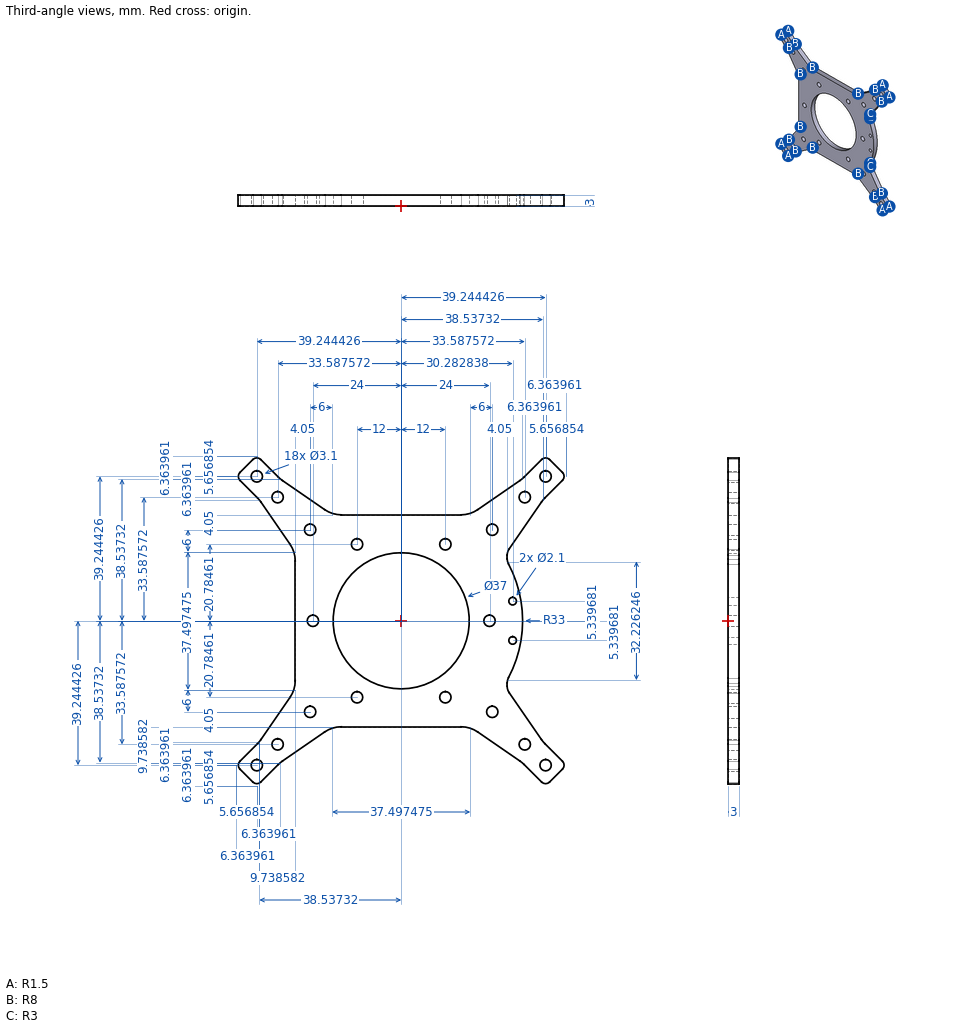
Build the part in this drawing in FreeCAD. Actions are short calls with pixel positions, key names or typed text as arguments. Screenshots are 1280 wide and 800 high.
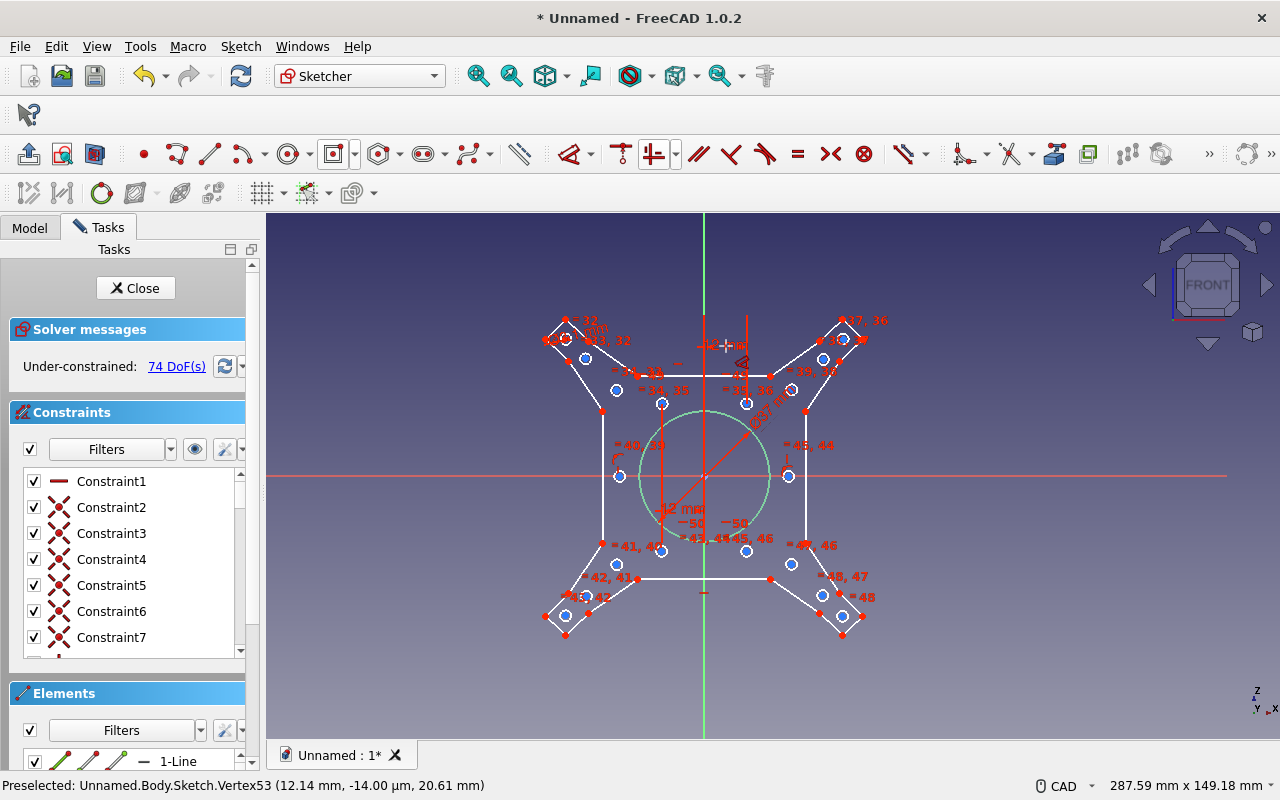
click(620, 476)
click(682, 442)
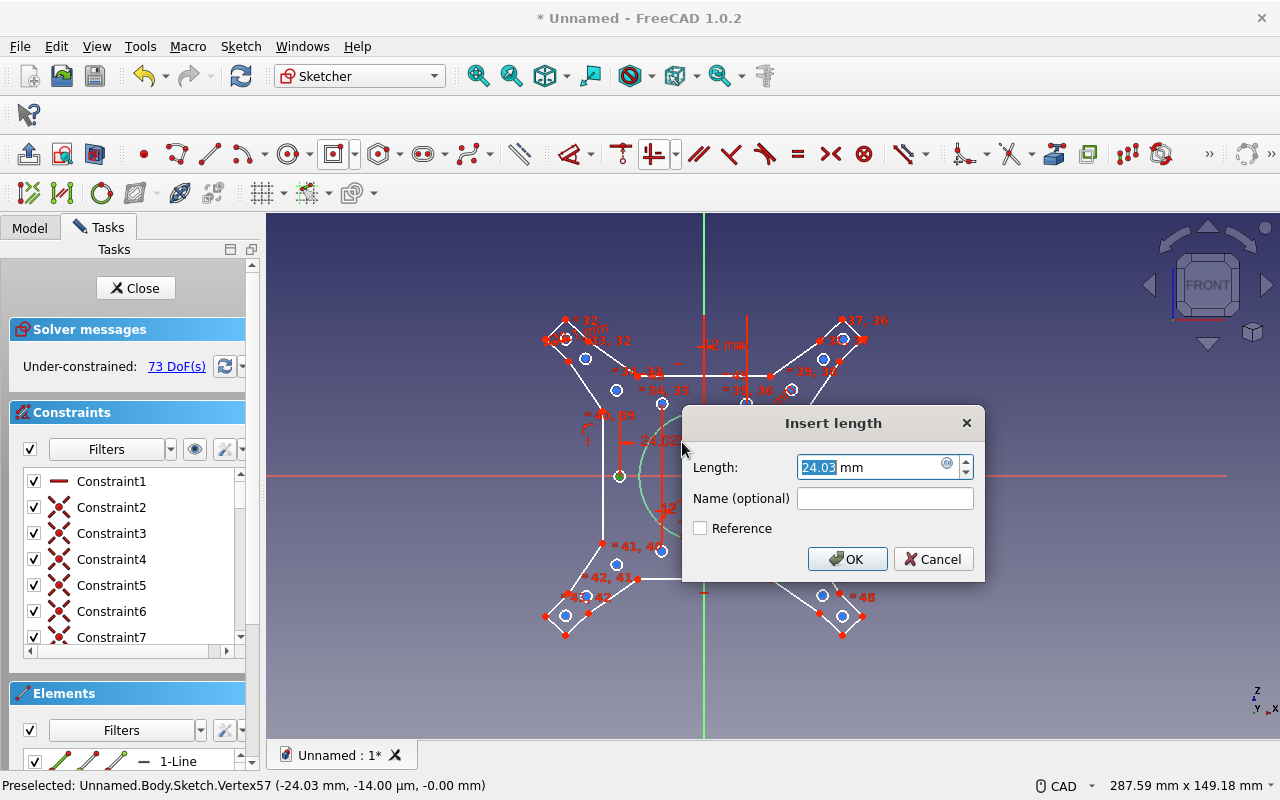
text(24)
key(Return)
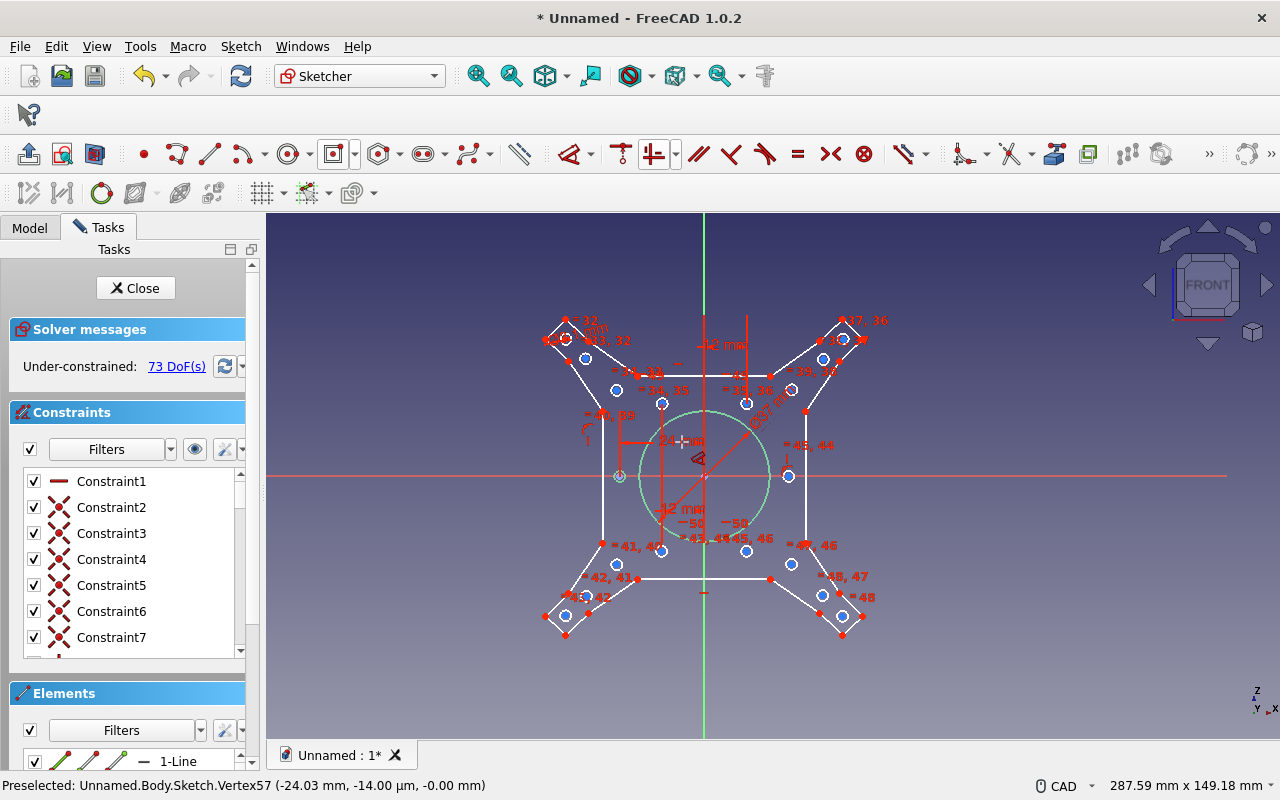
click(662, 551)
click(683, 609)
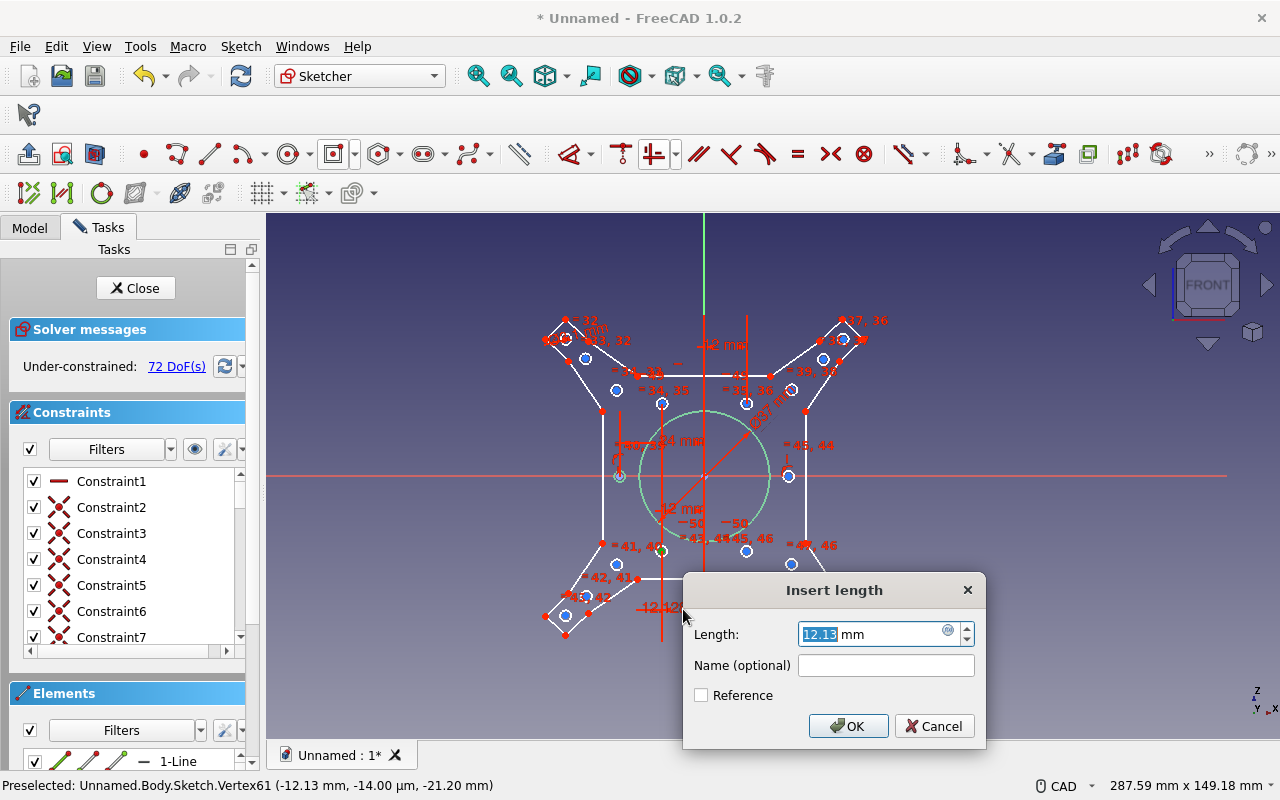
text(12)
key(Return)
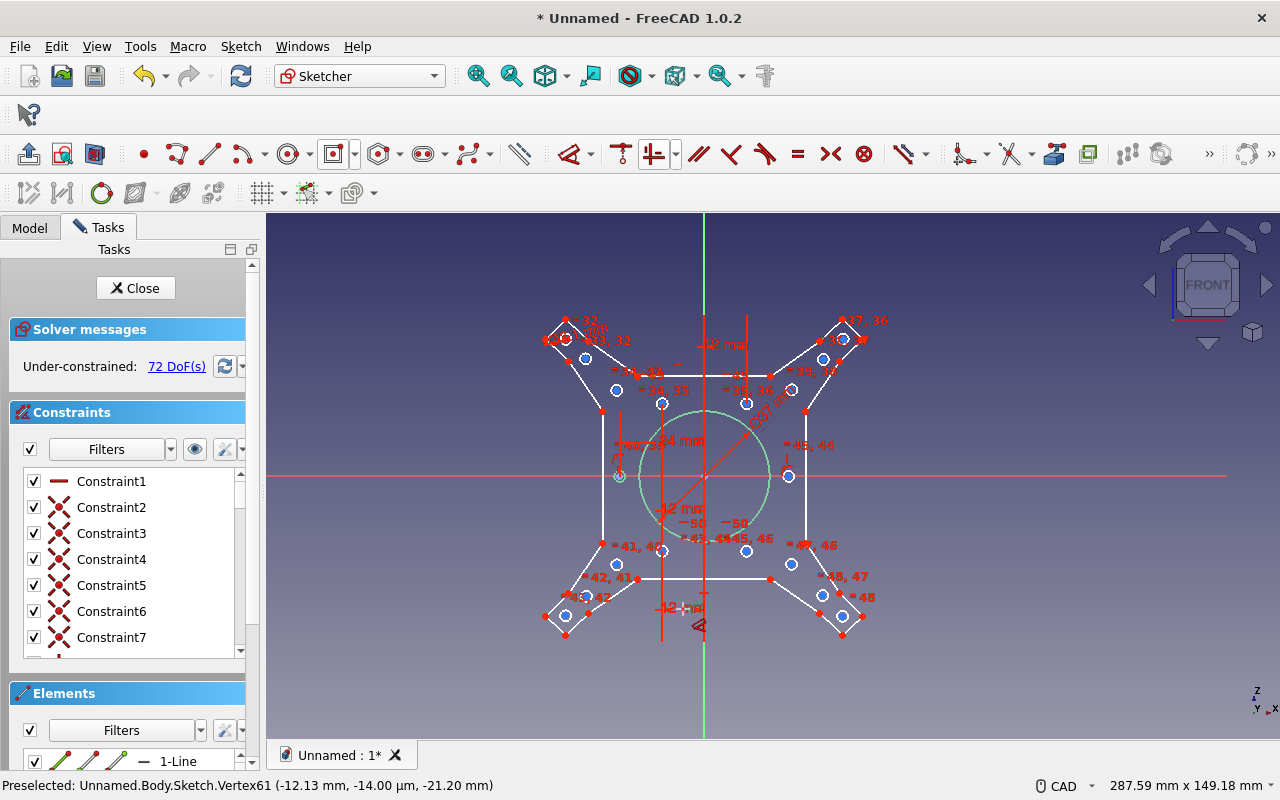
click(789, 476)
click(776, 510)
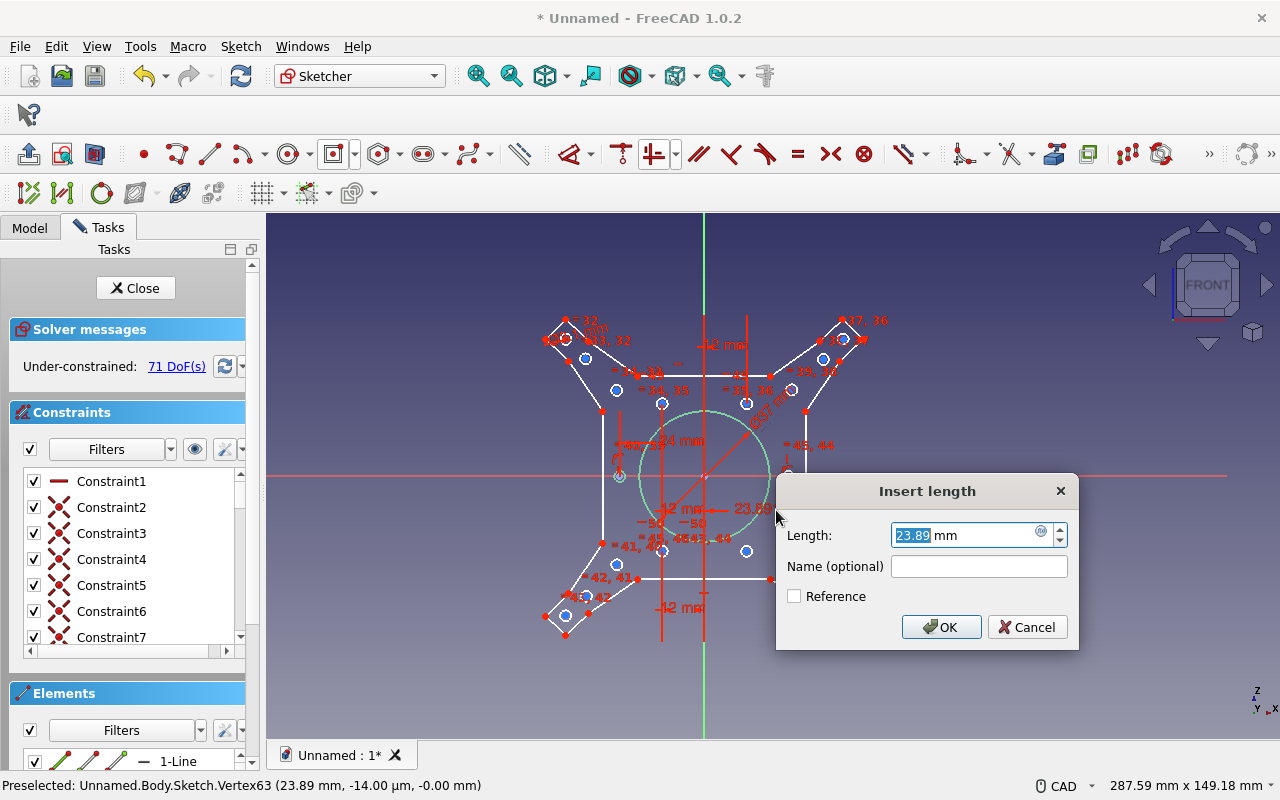
text(24)
key(Return)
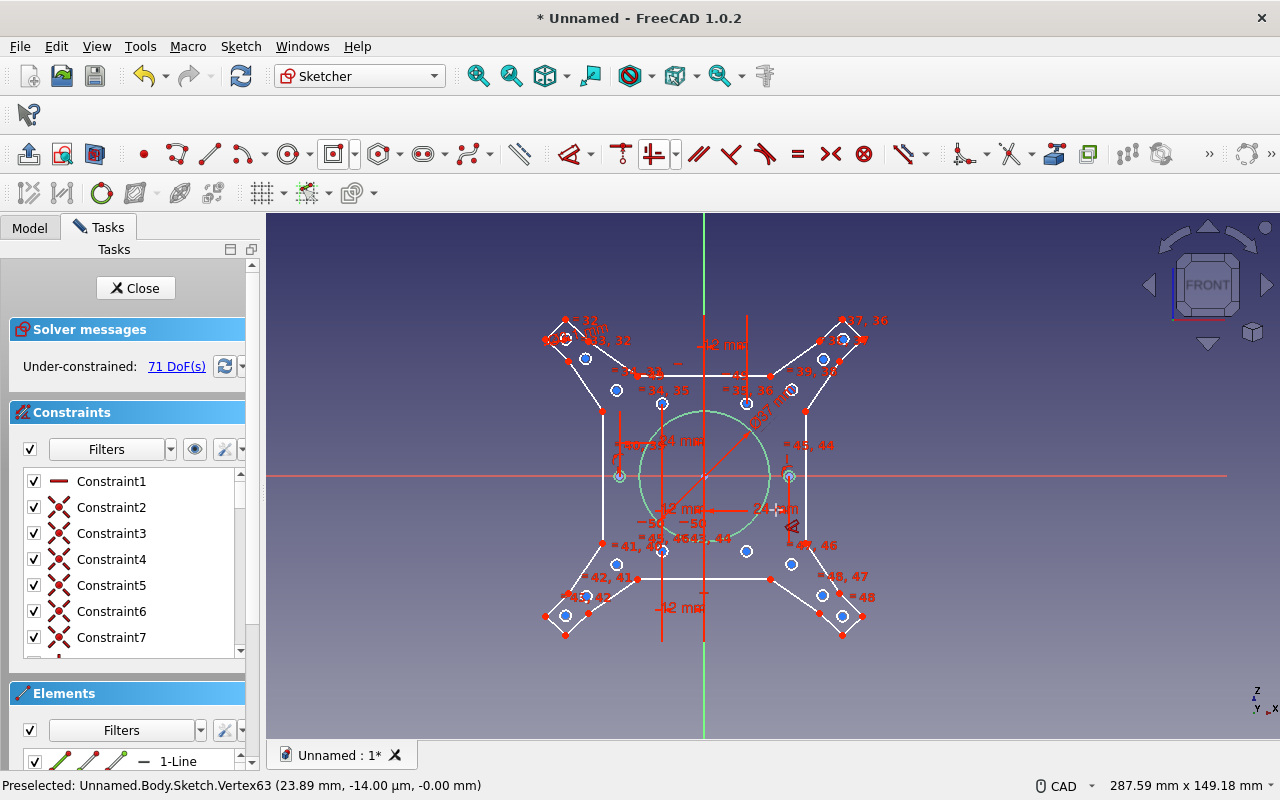
click(747, 551)
click(726, 633)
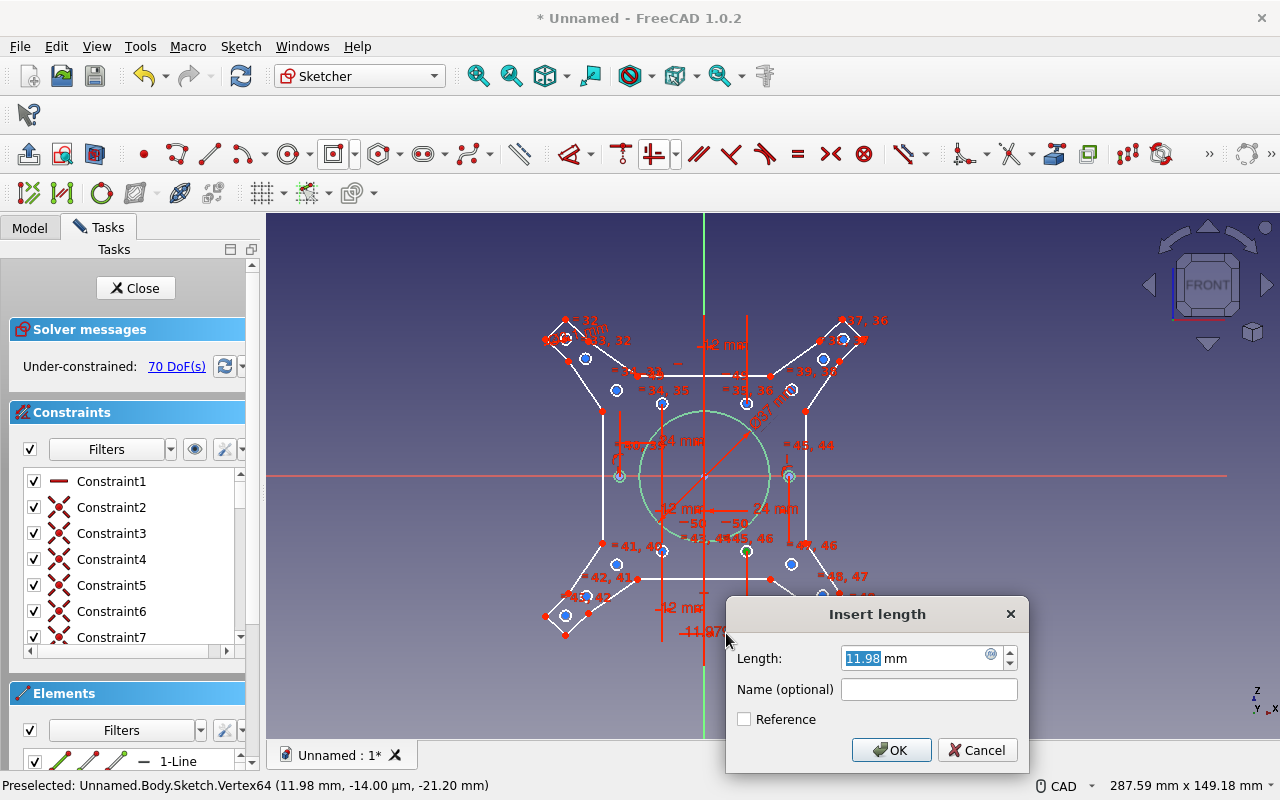
text(12)
key(Return)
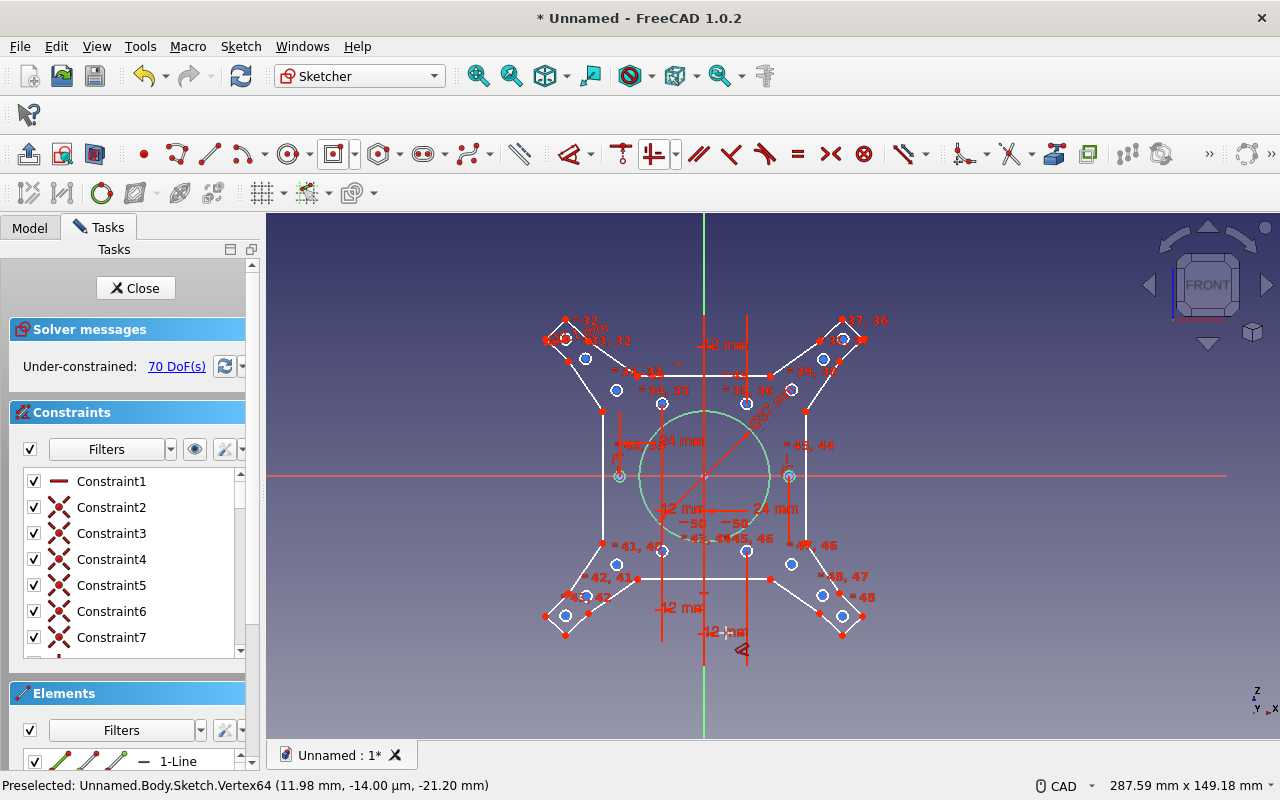
scroll(638, 376, up, 4)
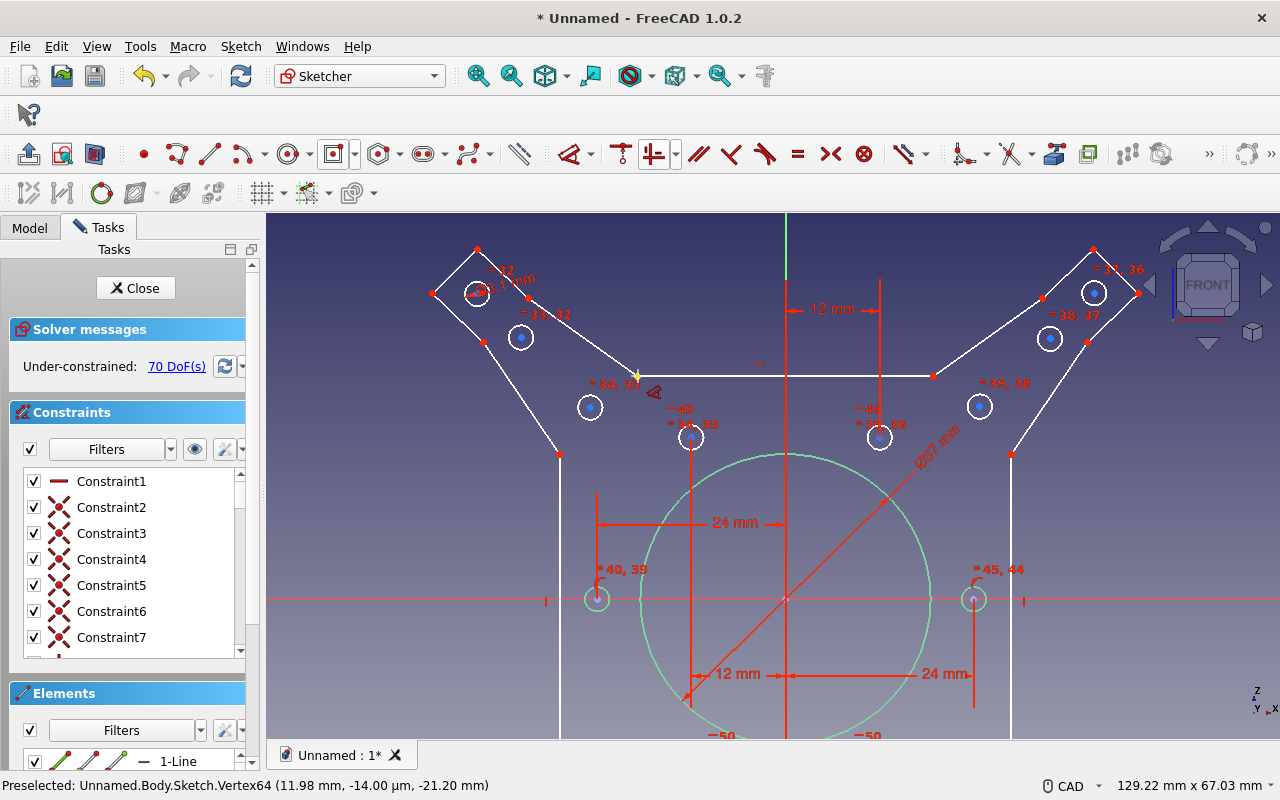
click(637, 376)